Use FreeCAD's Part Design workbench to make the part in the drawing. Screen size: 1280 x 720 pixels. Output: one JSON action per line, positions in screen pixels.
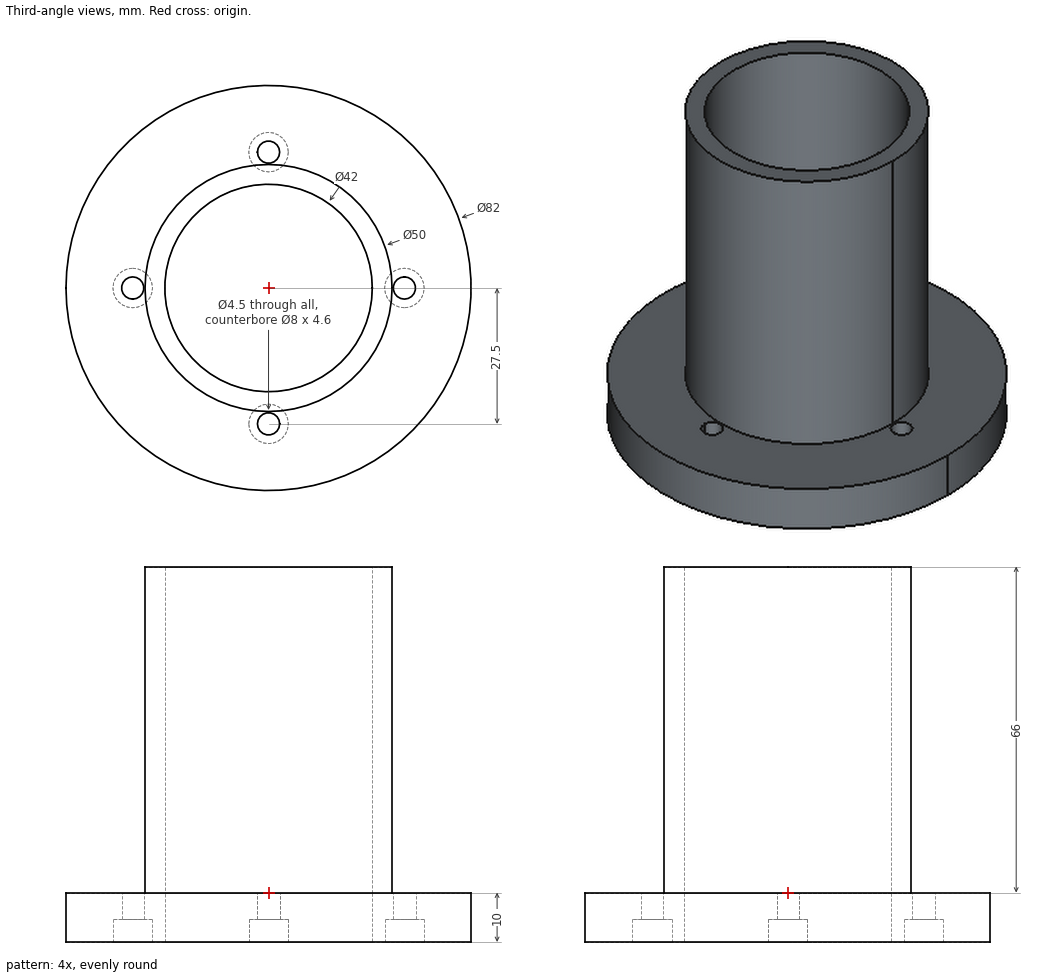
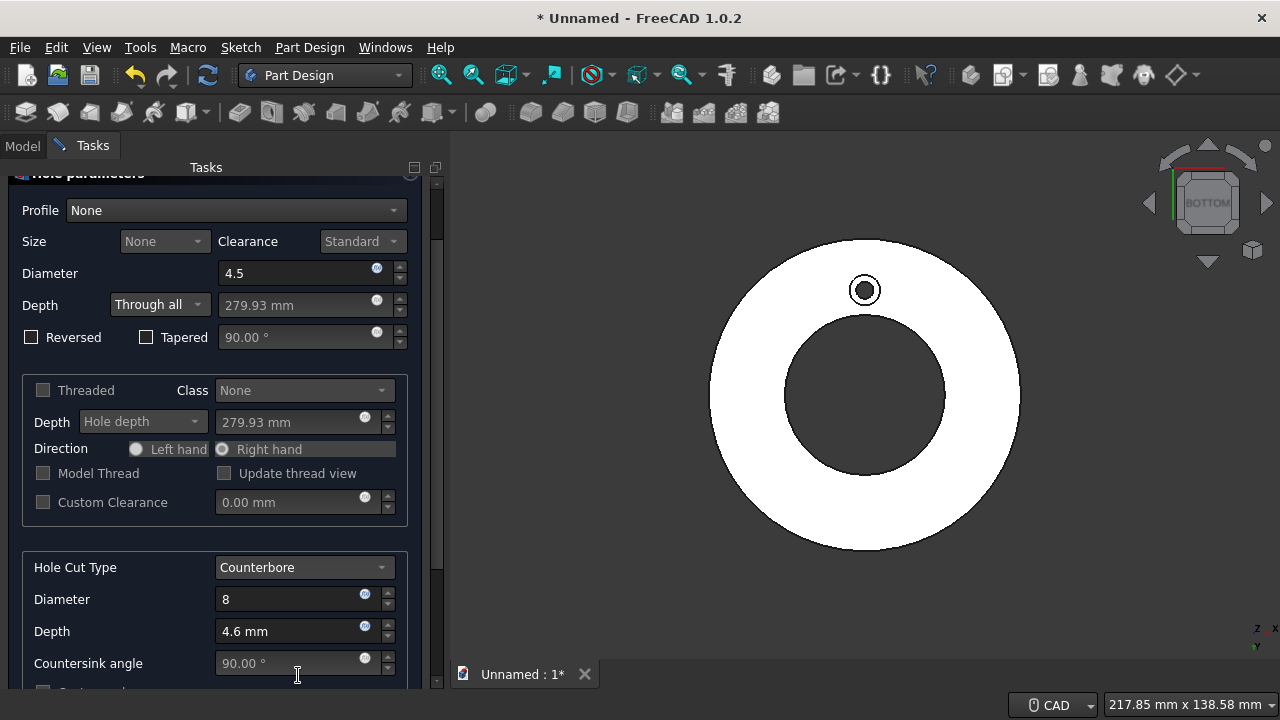
{"action": "scroll", "coordinate": [437, 432], "scroll_direction": "up", "scroll_amount": 3}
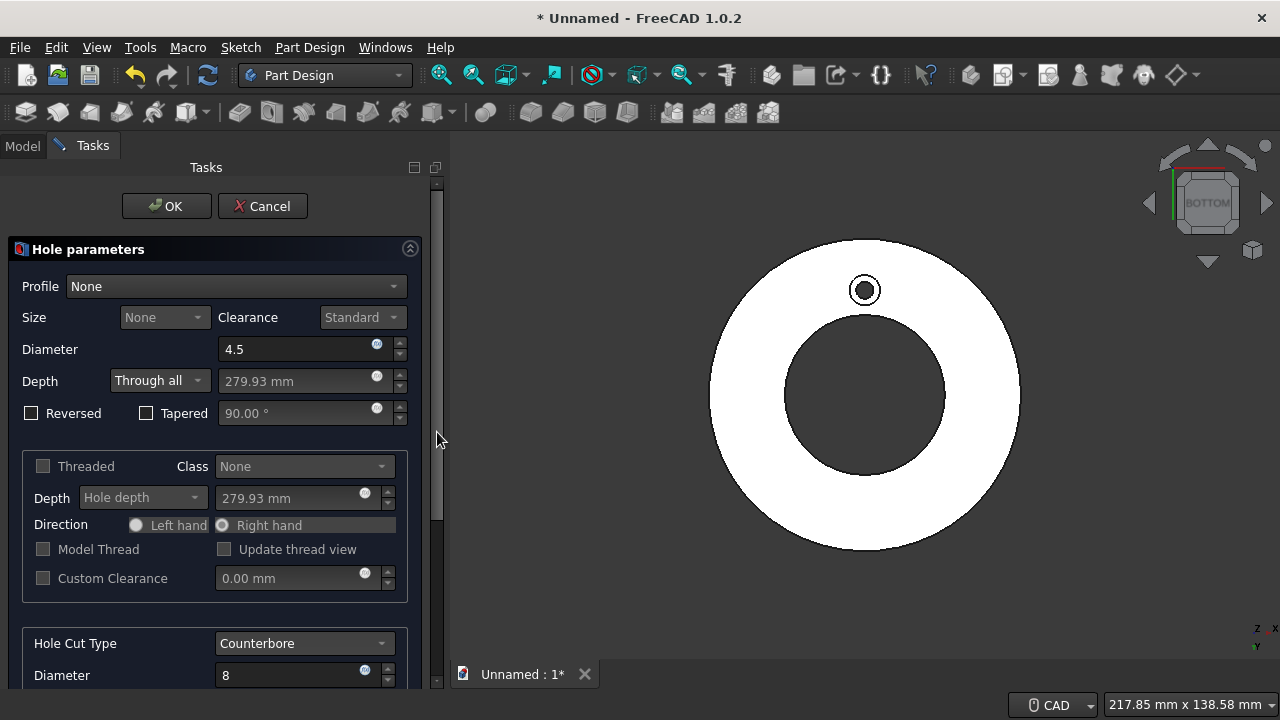
{"action": "left_click", "coordinate": [167, 206]}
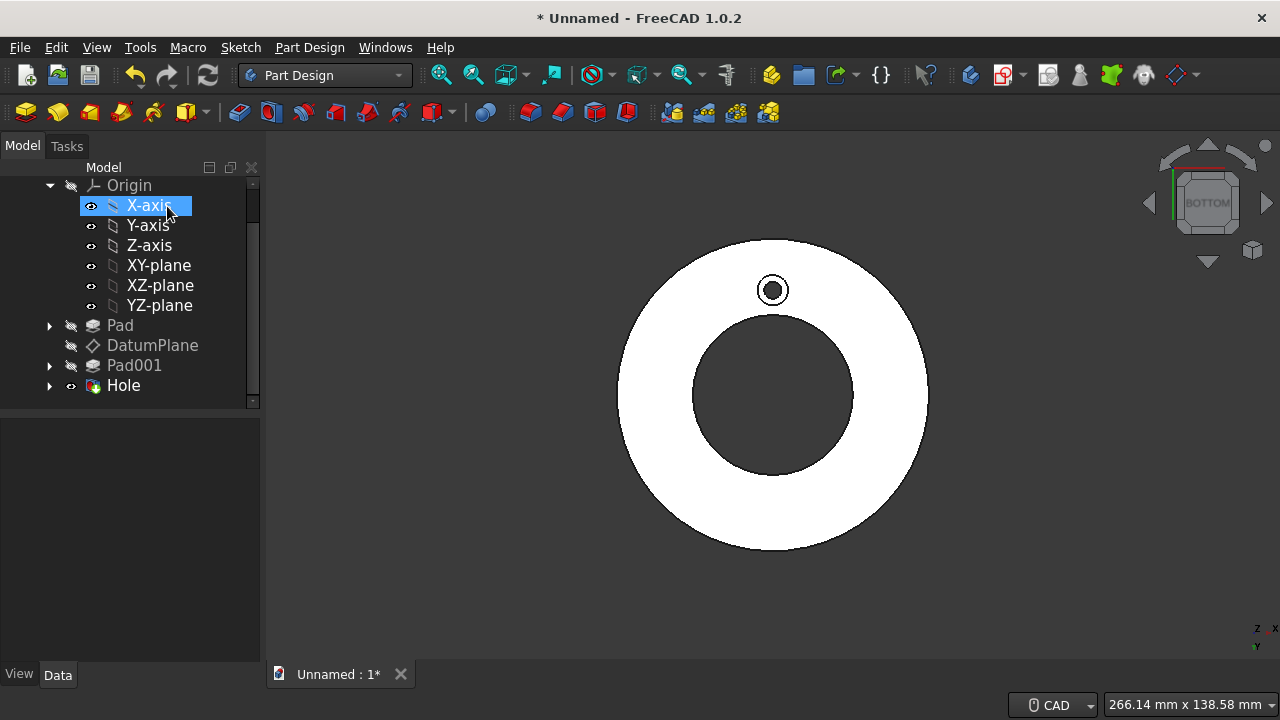
{"action": "left_click", "coordinate": [116, 386]}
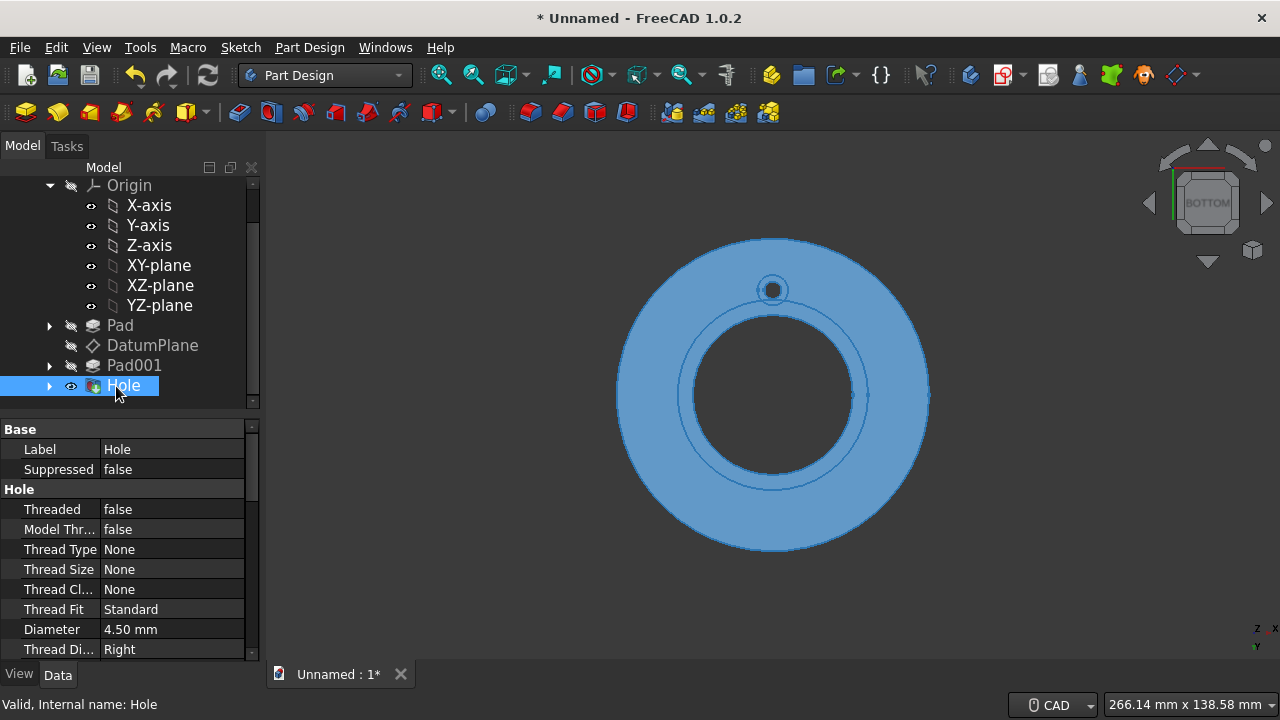
{"action": "left_click", "coordinate": [736, 112]}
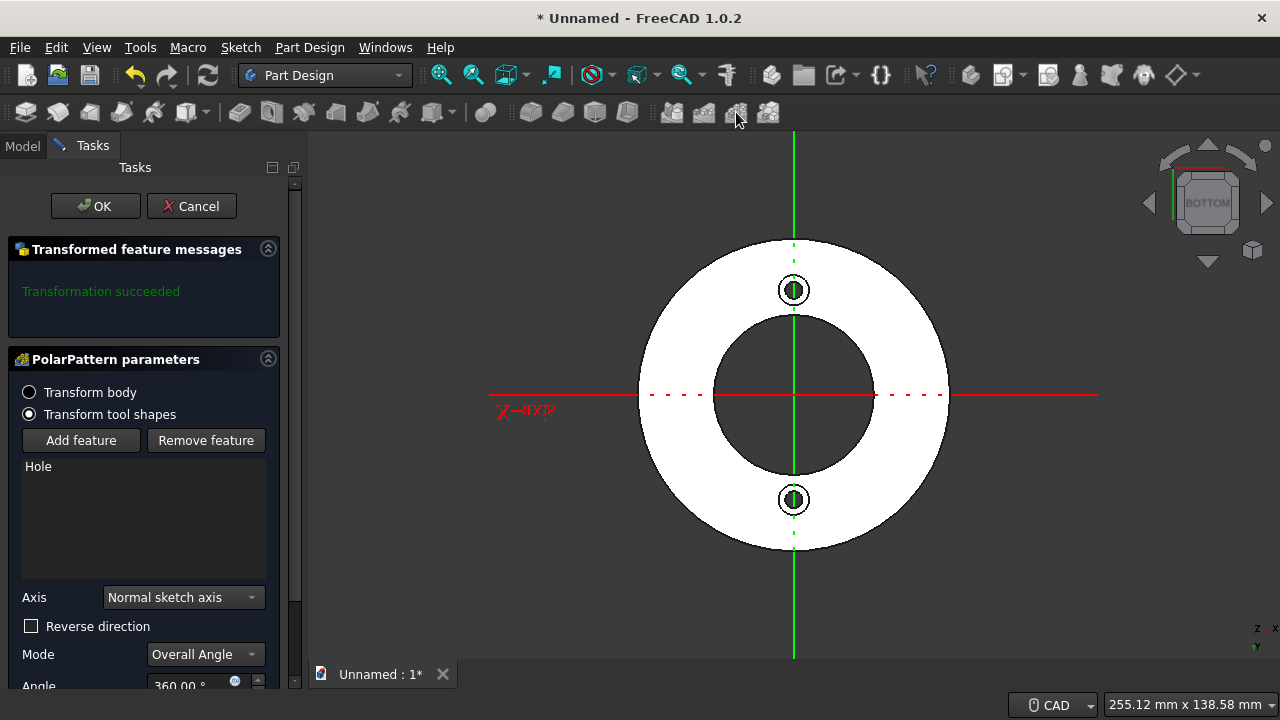
{"action": "left_click", "coordinate": [184, 598]}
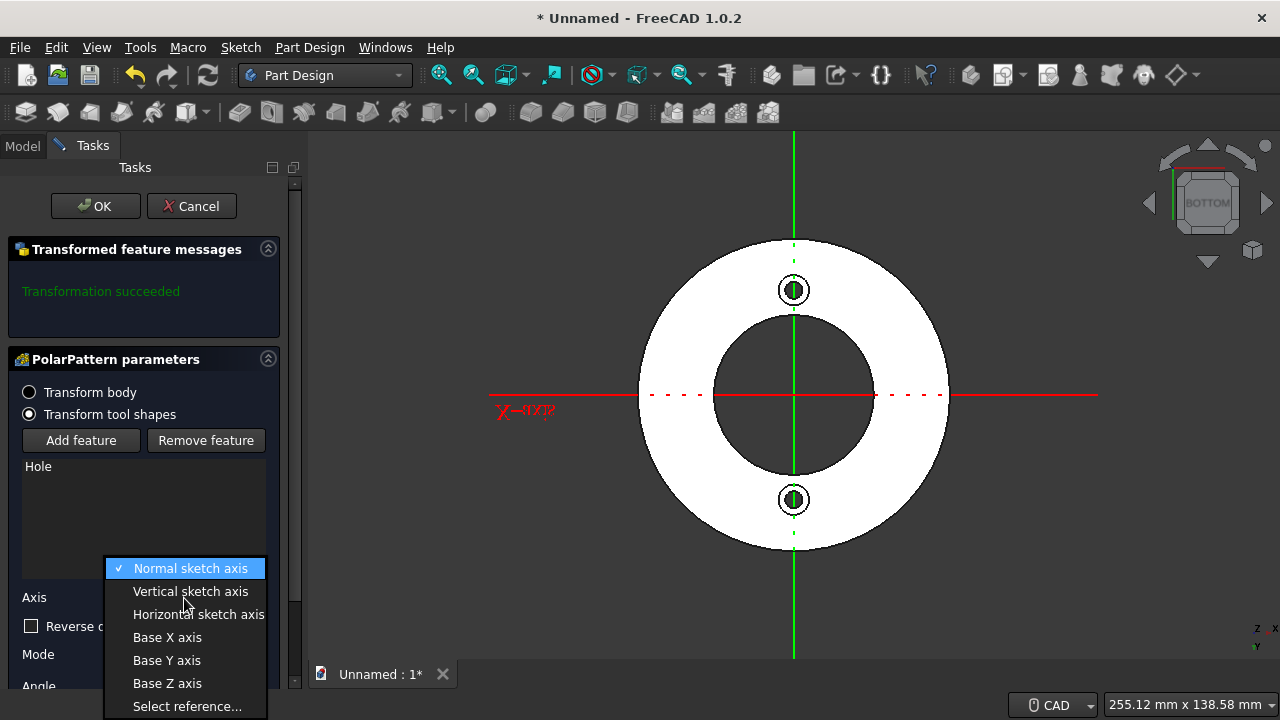
{"action": "left_click", "coordinate": [184, 684]}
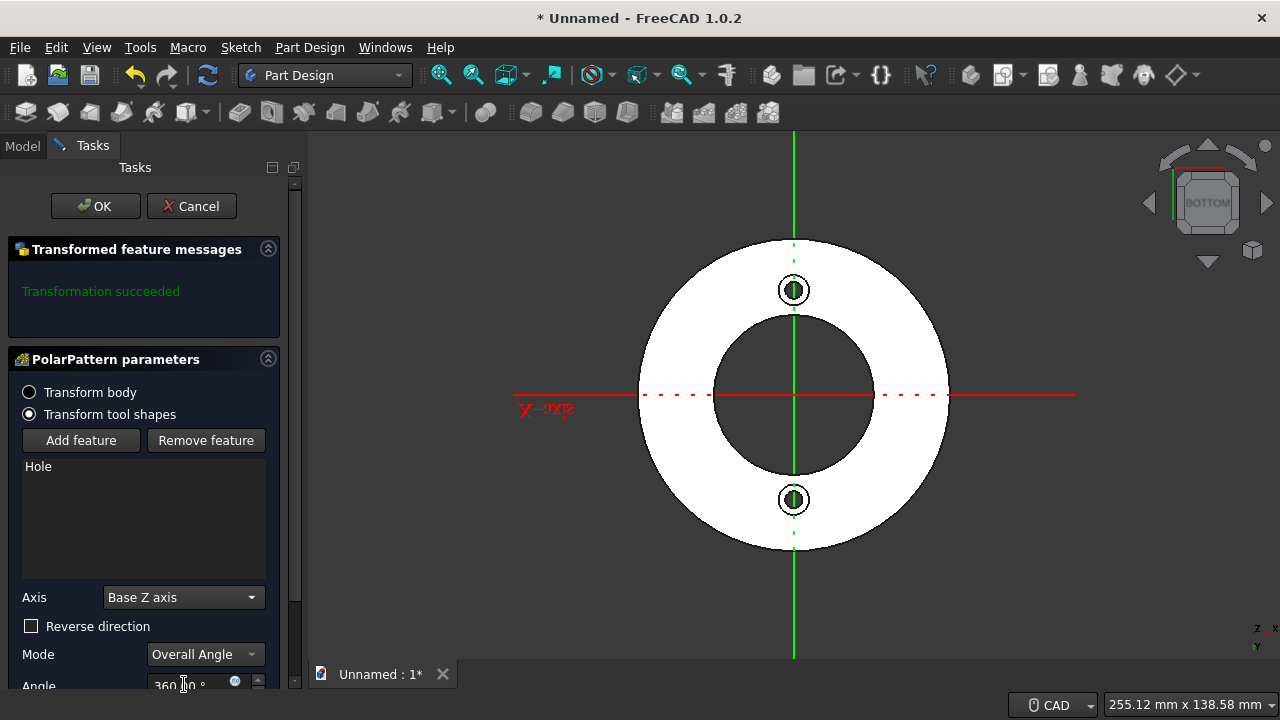
{"action": "scroll", "coordinate": [295, 432], "scroll_direction": "down", "scroll_amount": 2}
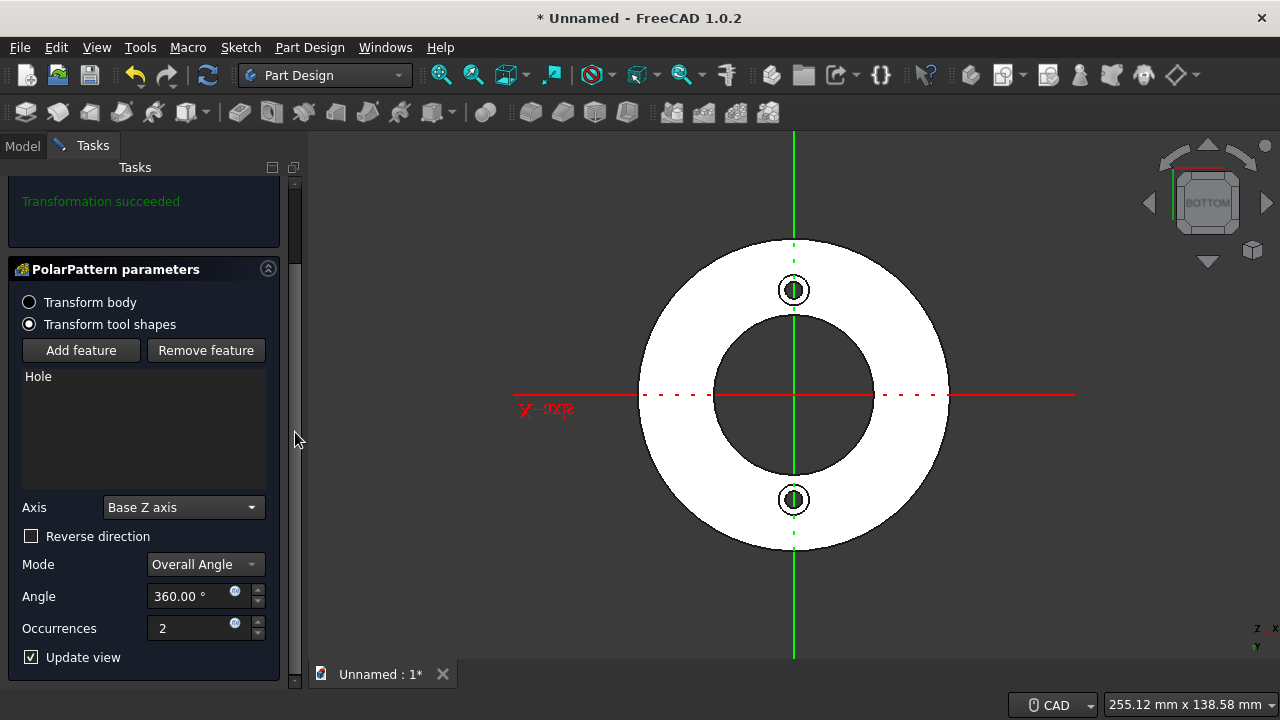
{"action": "triple_click", "coordinate": [198, 628]}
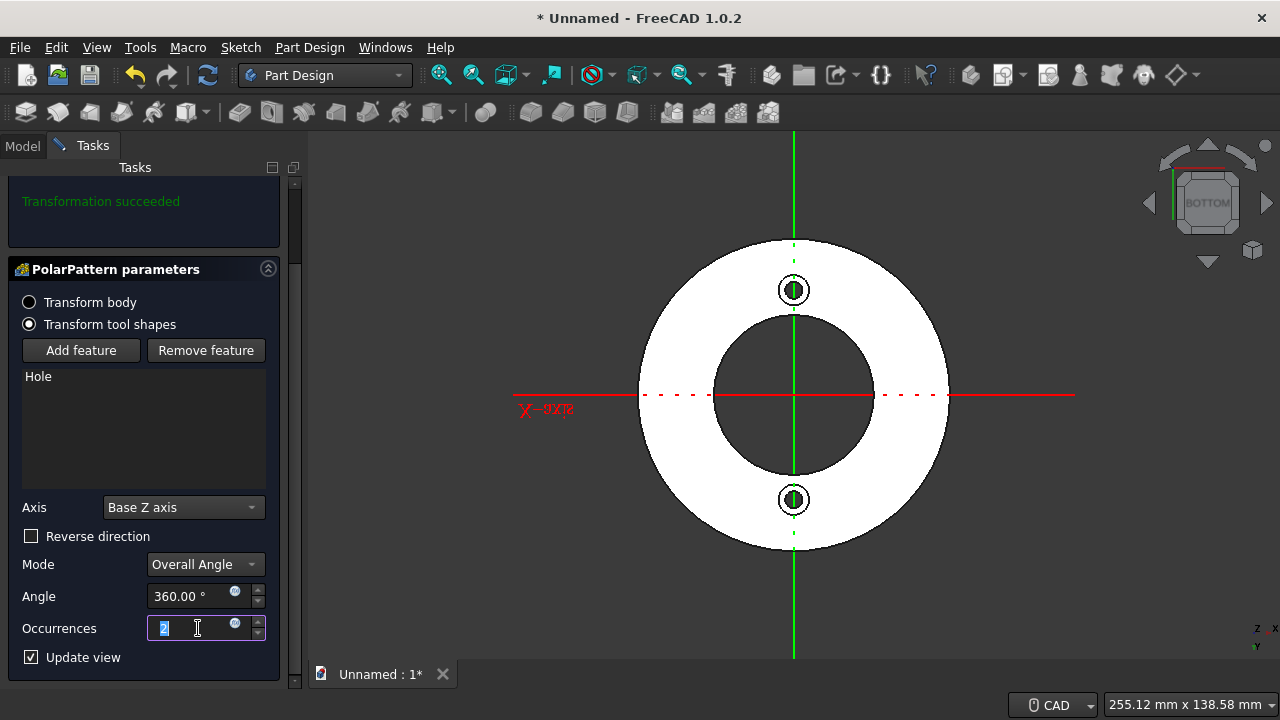
{"action": "type", "text": "4"}
{"action": "key", "text": "Tab"}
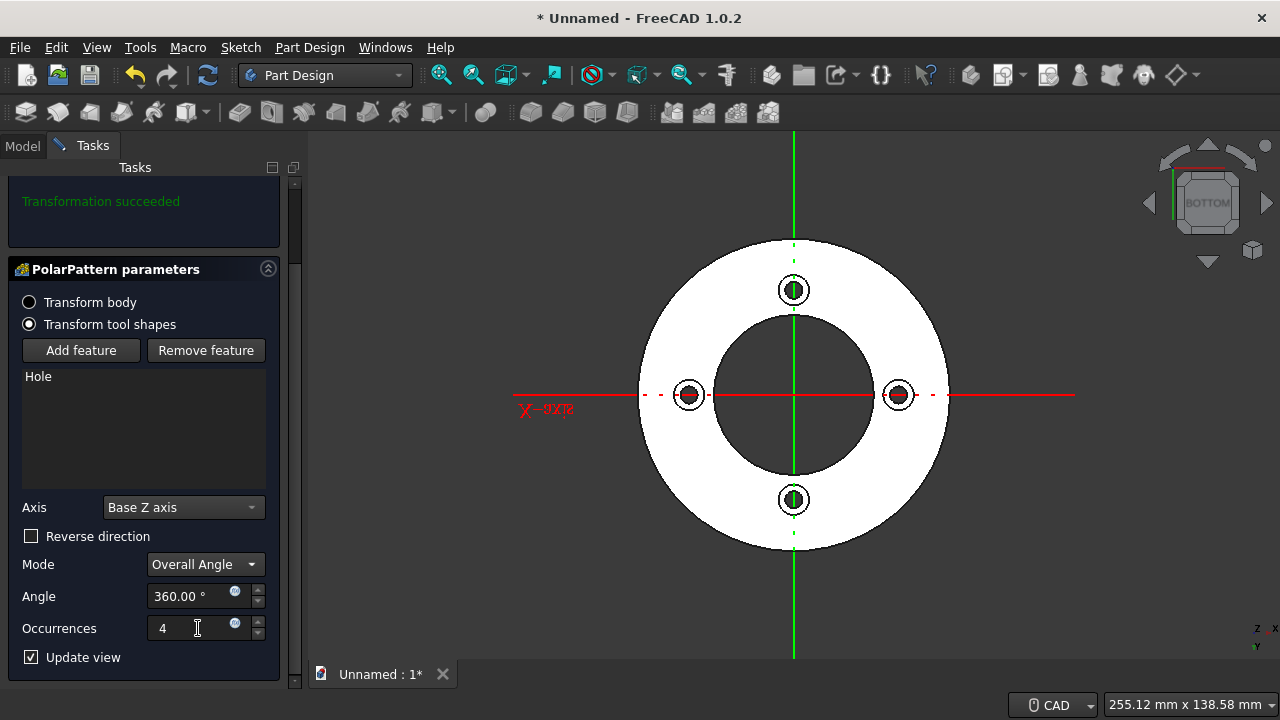
{"action": "scroll", "coordinate": [295, 432], "scroll_direction": "up", "scroll_amount": 3}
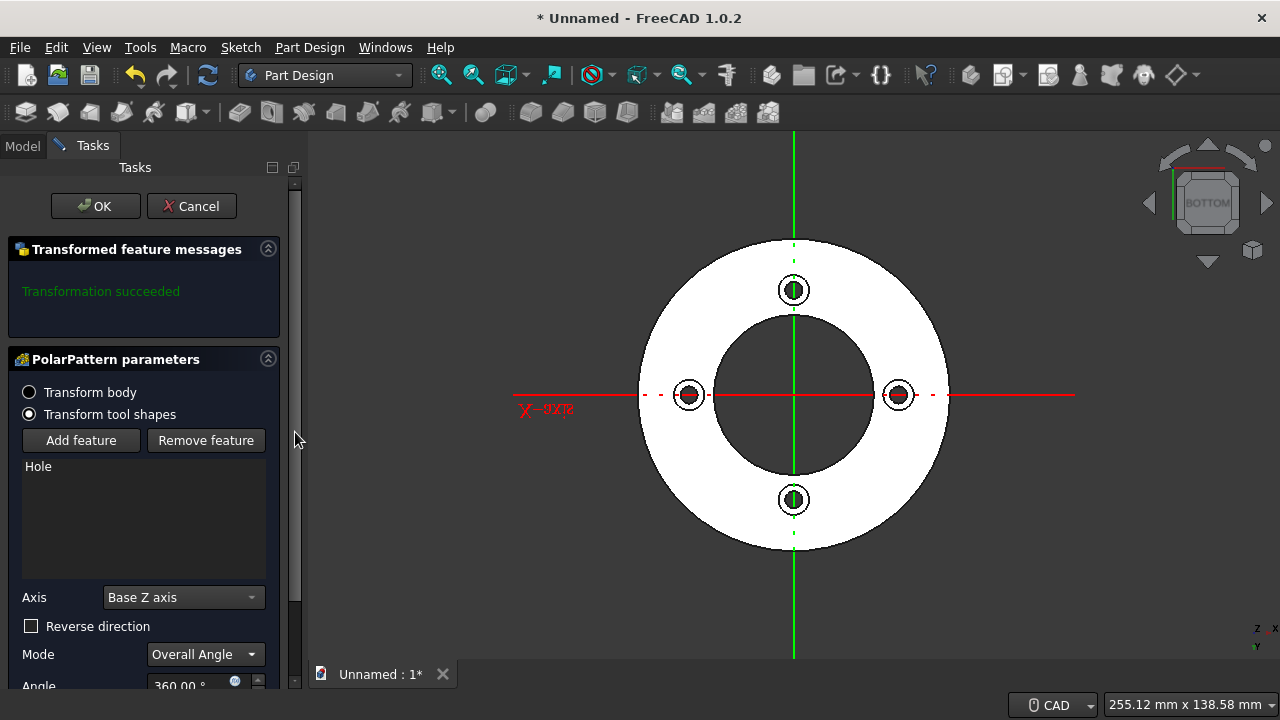
{"action": "left_click", "coordinate": [96, 206]}